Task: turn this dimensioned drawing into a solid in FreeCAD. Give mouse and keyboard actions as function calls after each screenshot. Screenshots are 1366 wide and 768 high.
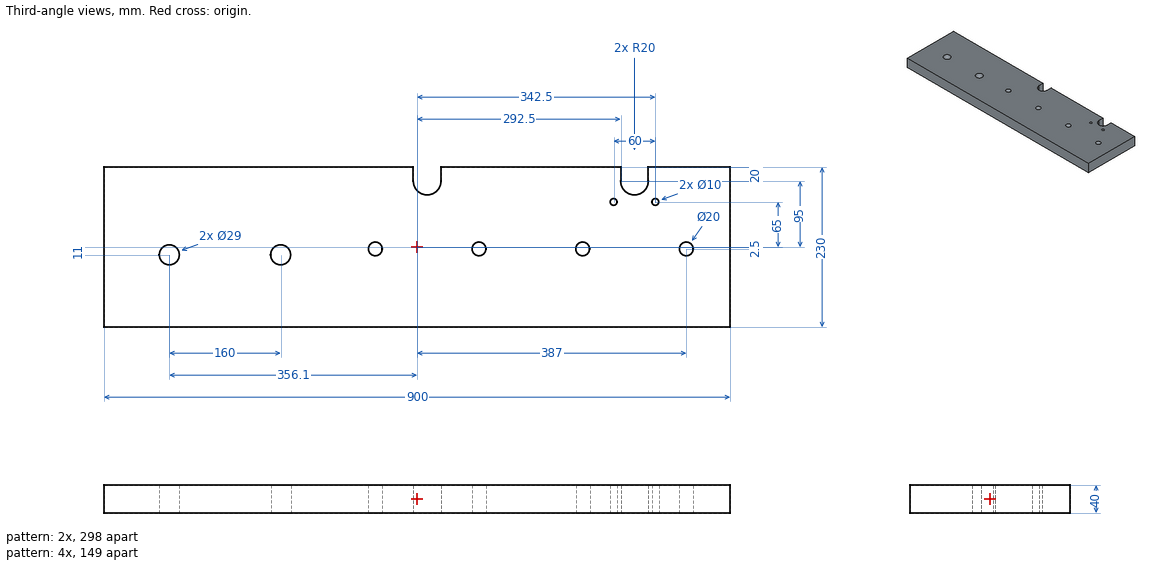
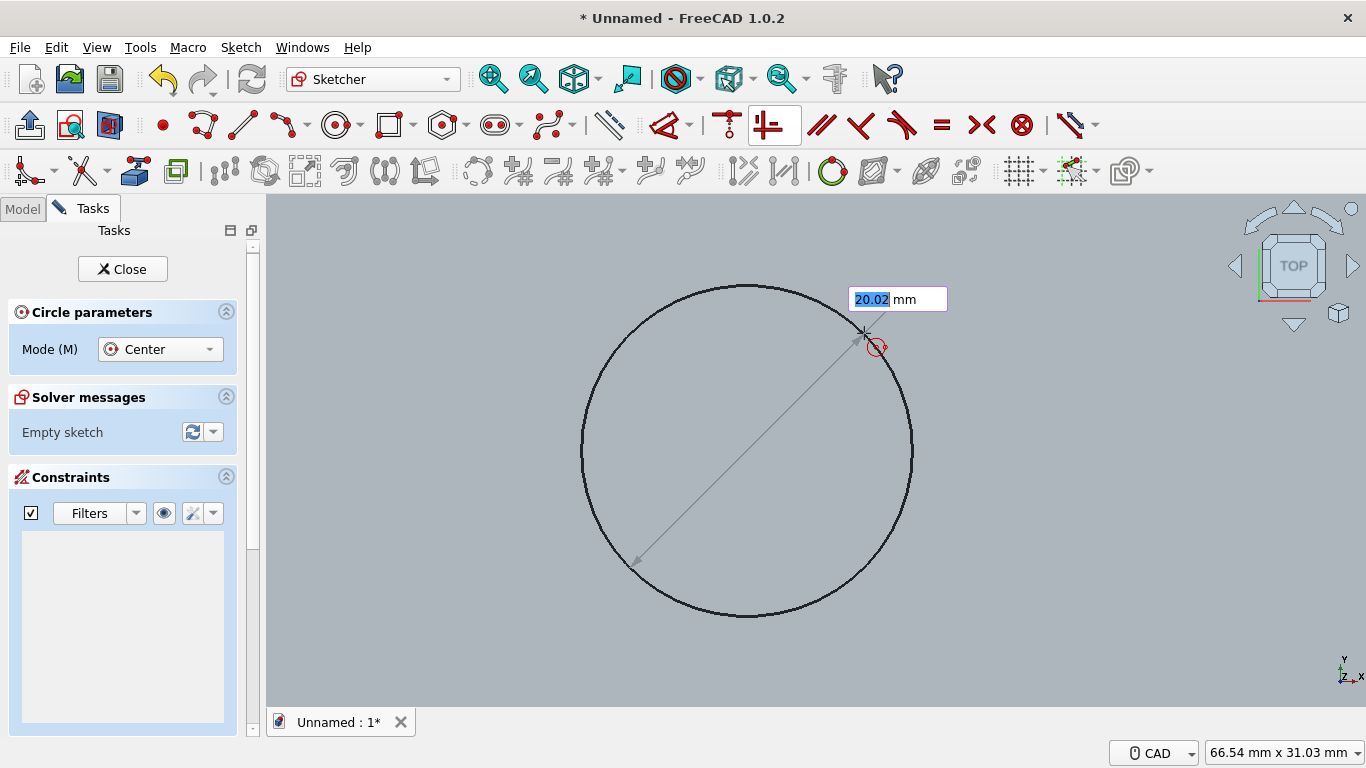
text(20)
key(Return)
key(Escape)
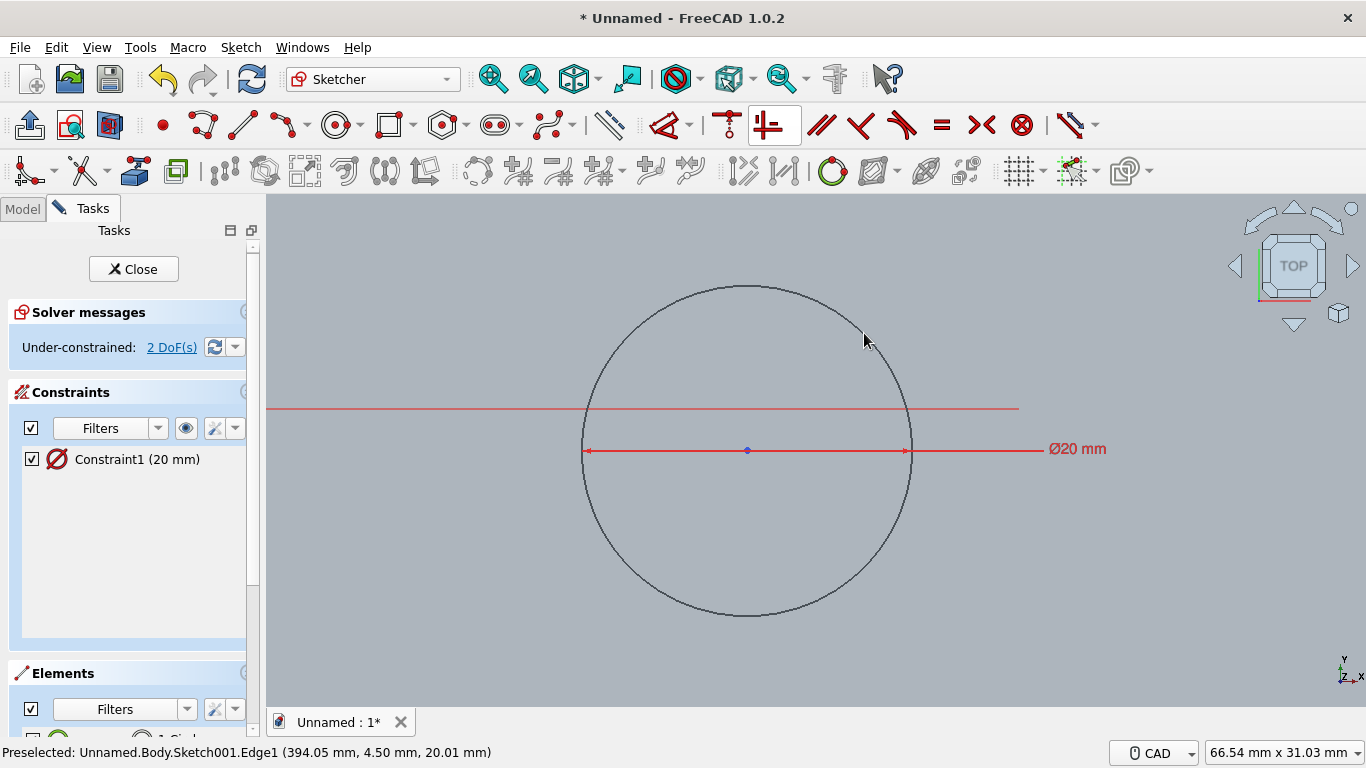
click(747, 451)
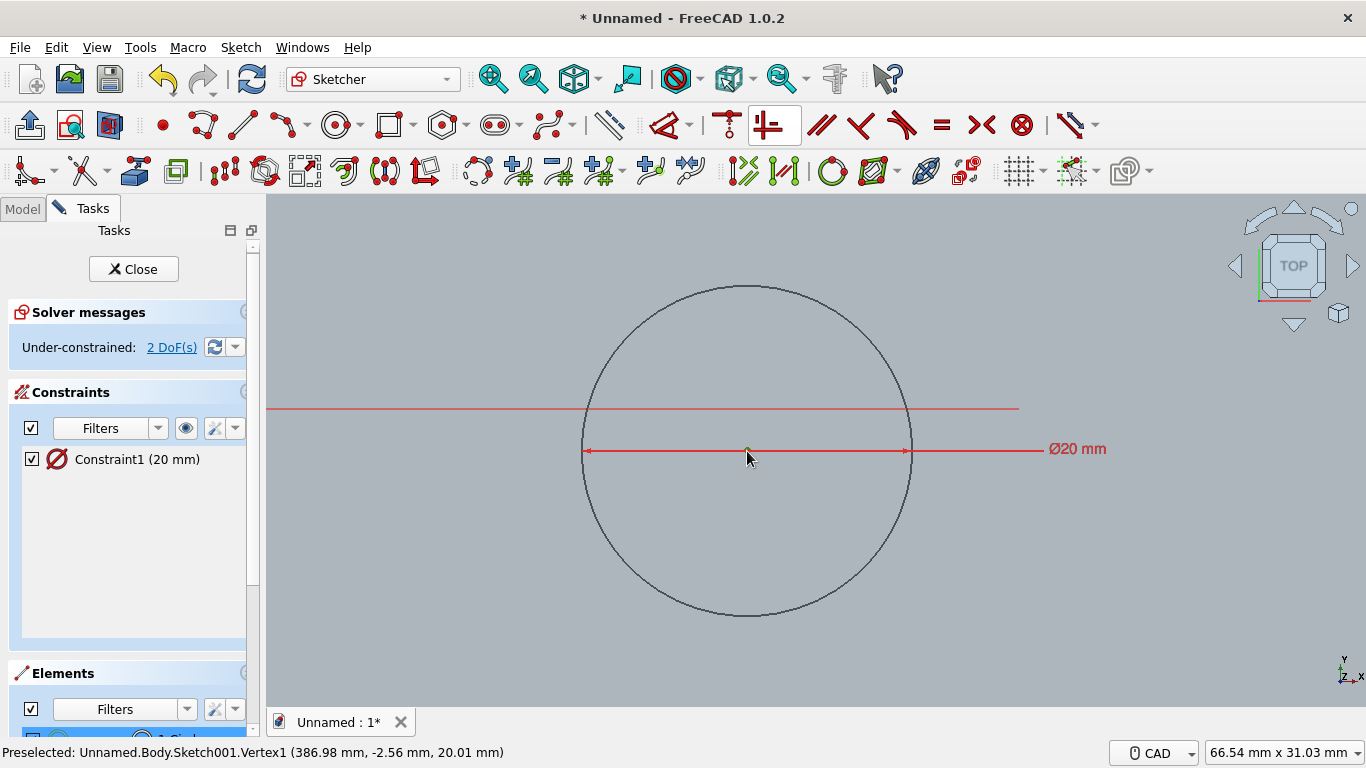
click(692, 126)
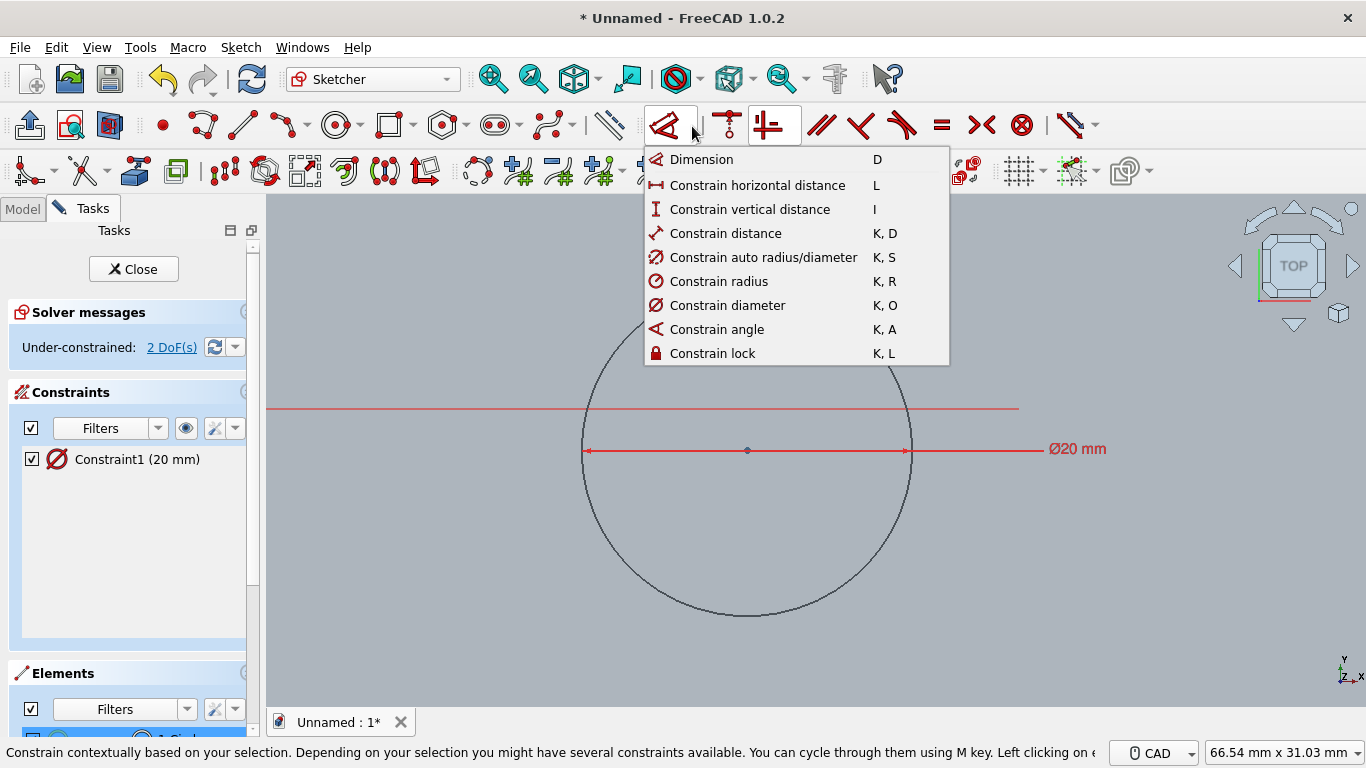
click(797, 185)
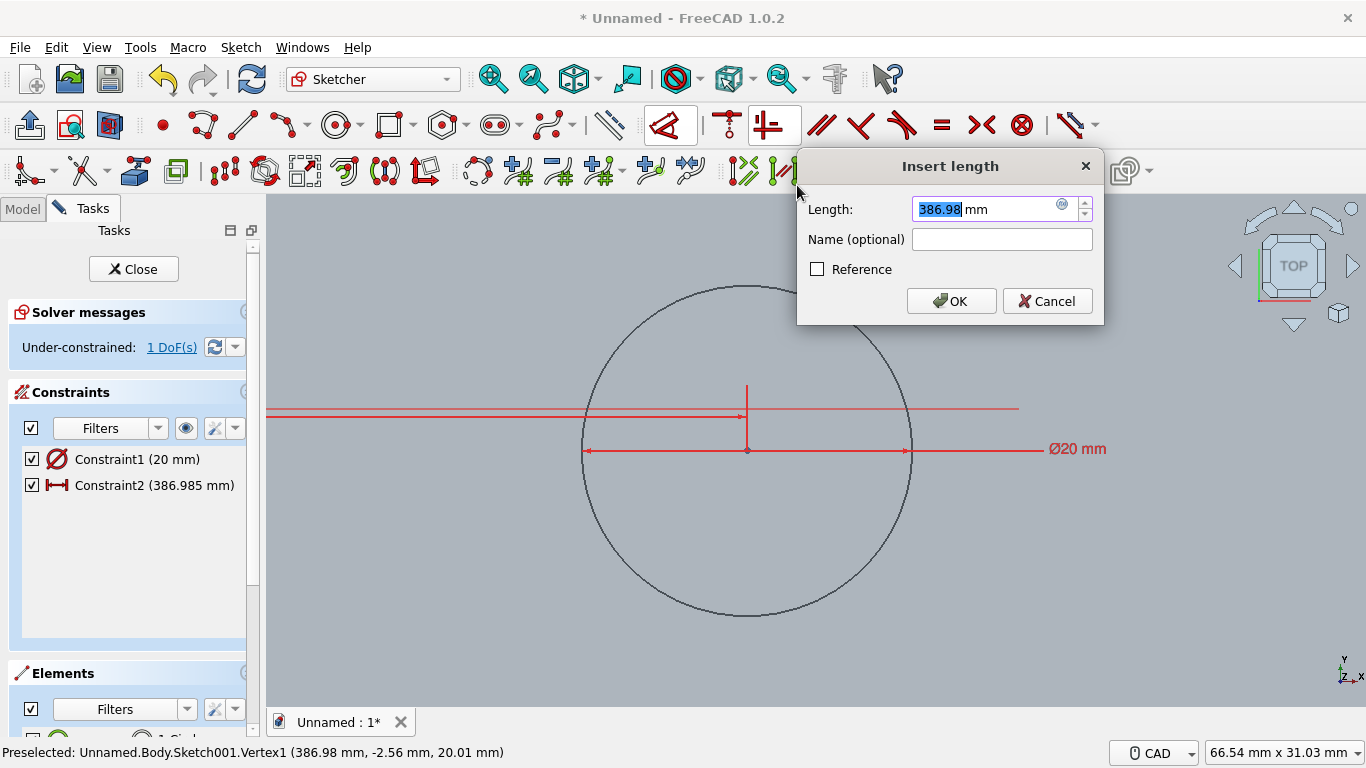
text(387)
key(Return)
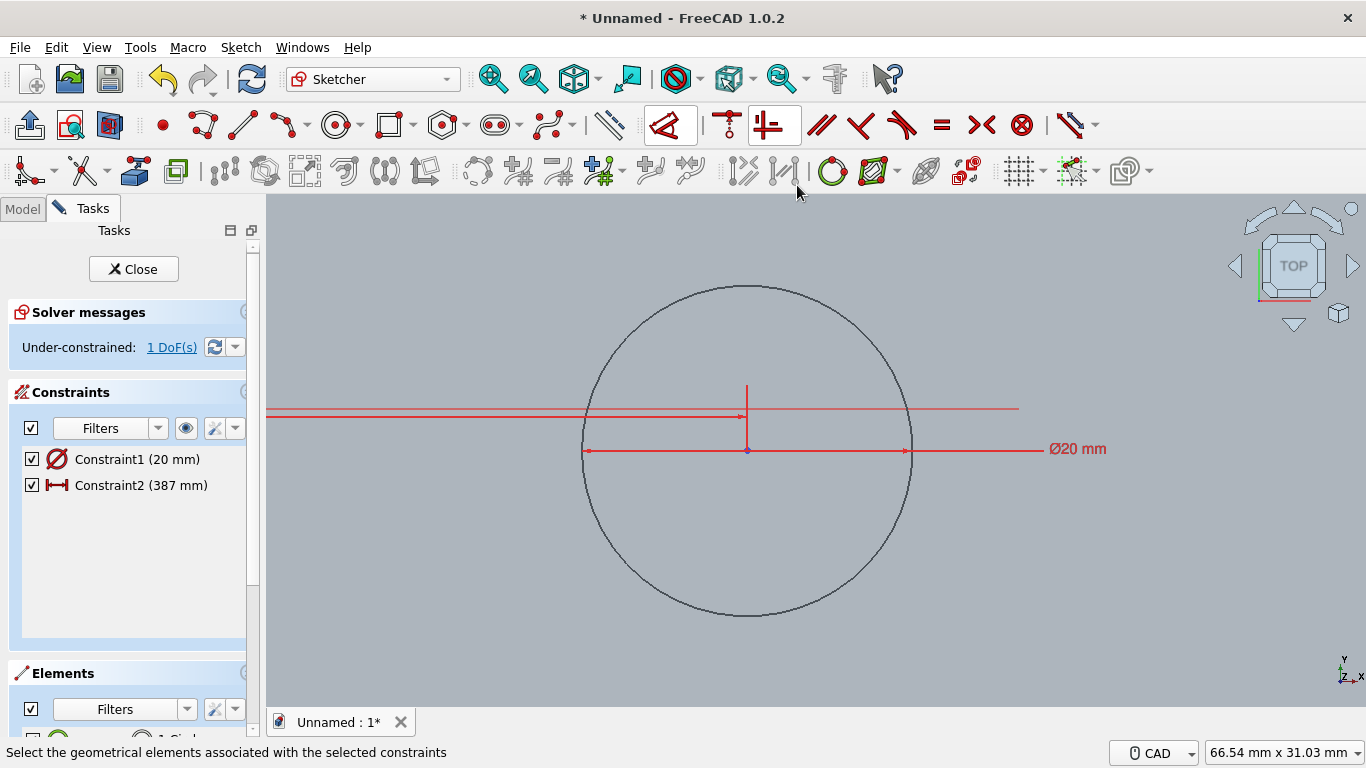
click(747, 451)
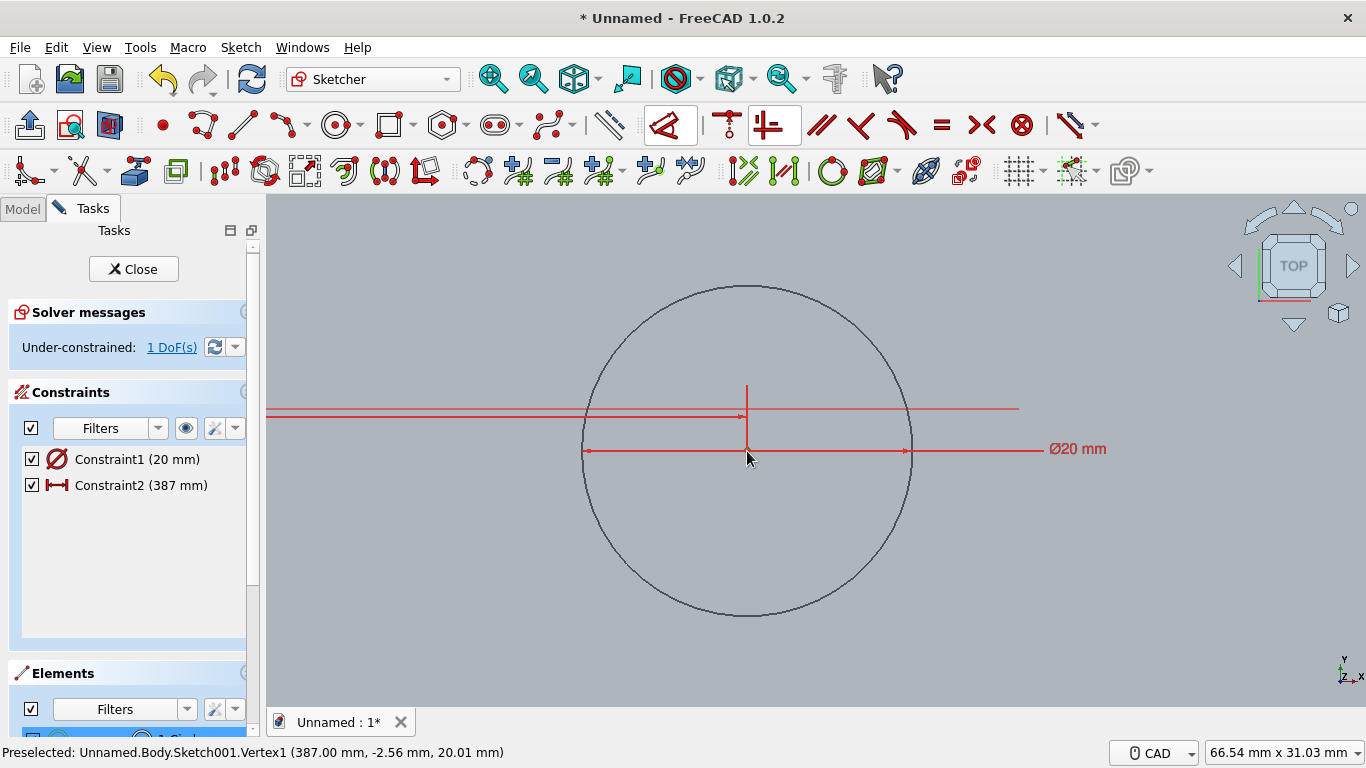
key(i)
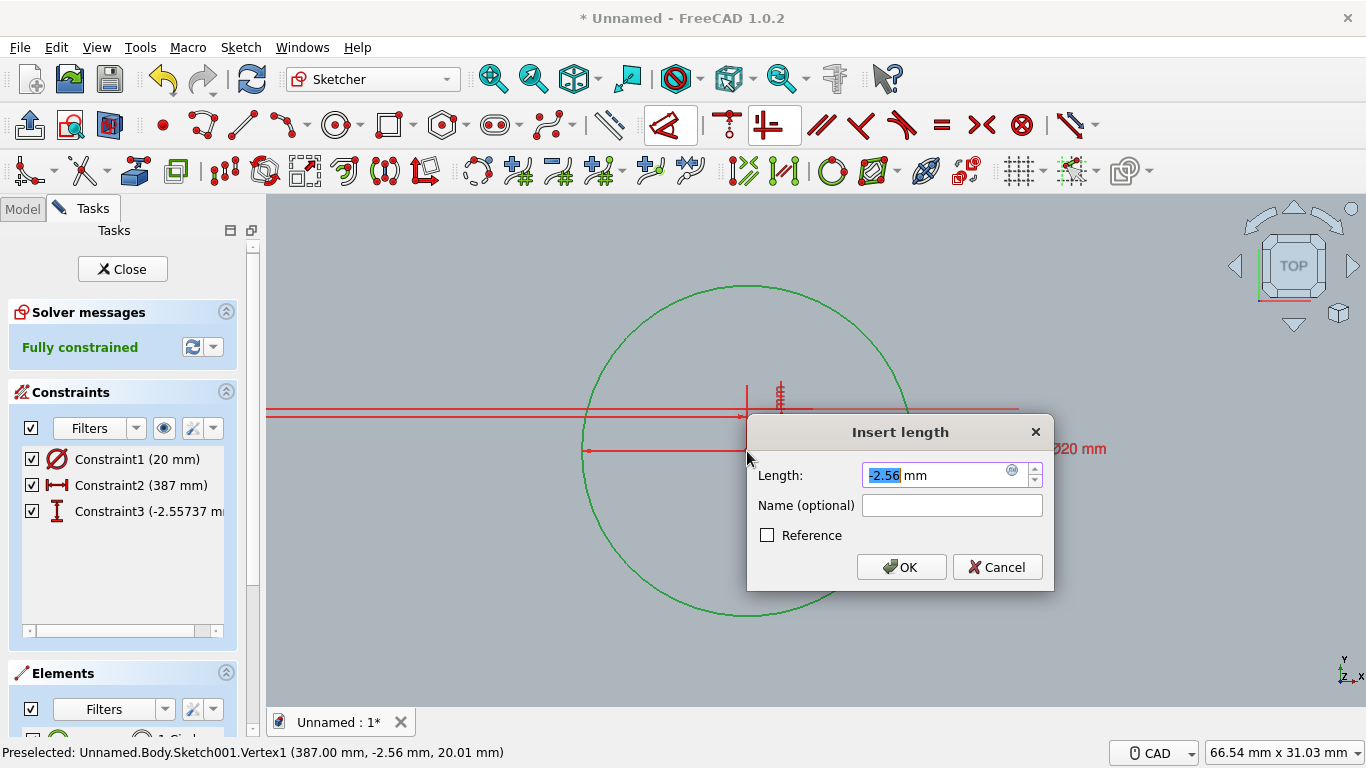
text(-2.5)
key(Return)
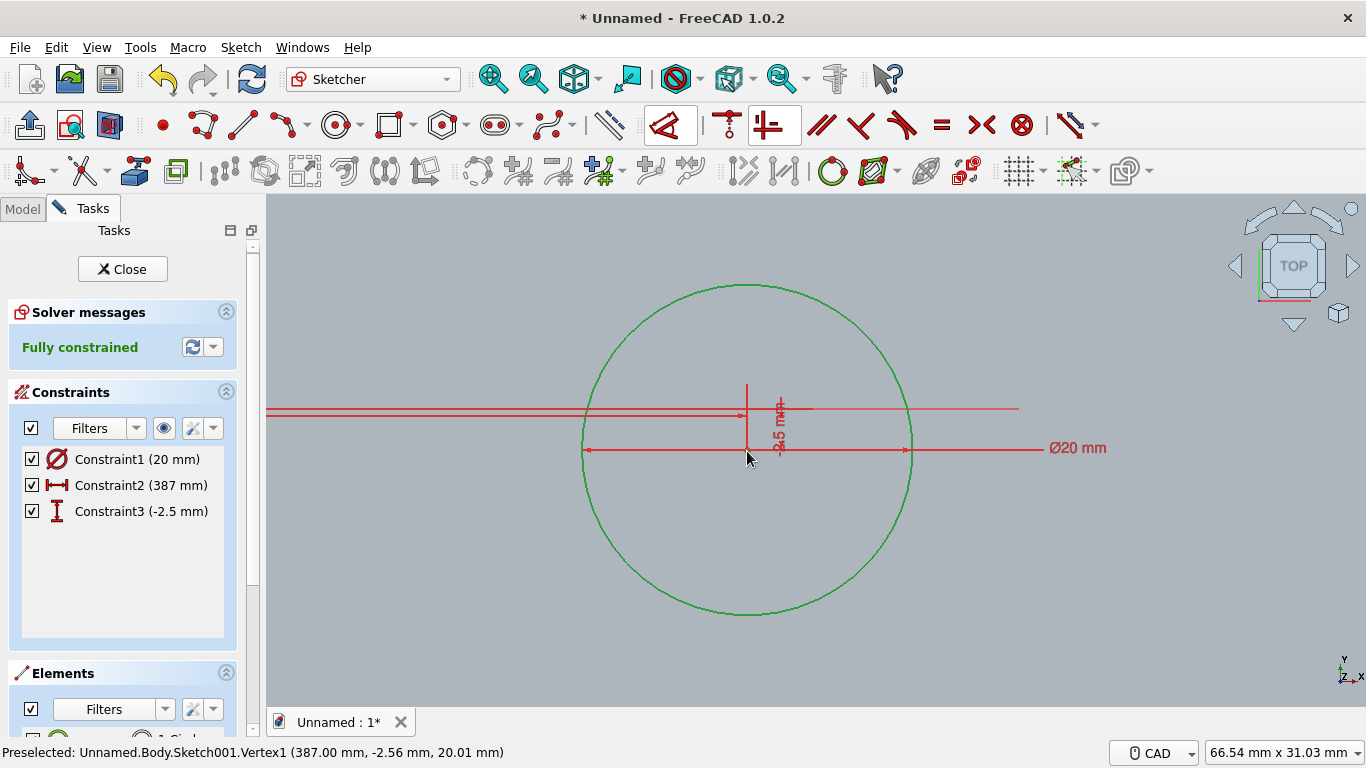
click(123, 269)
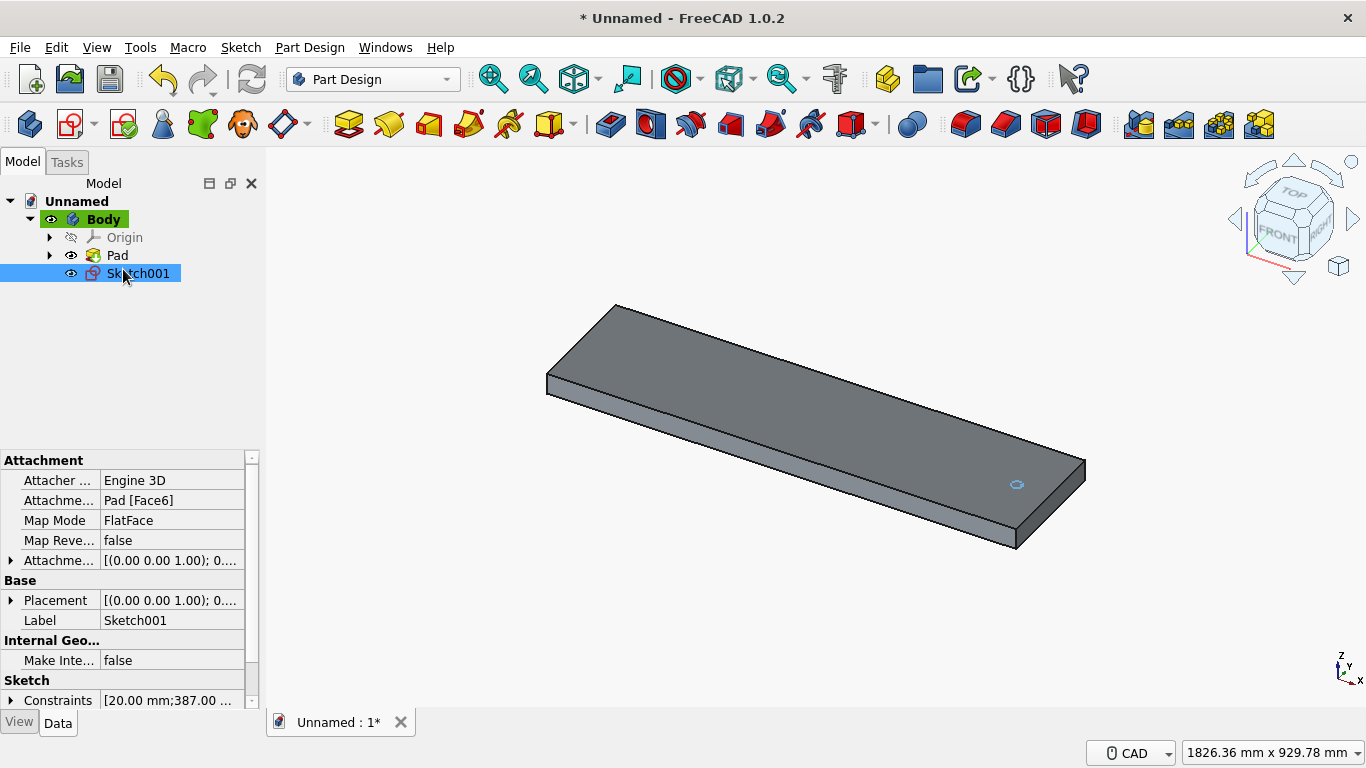
click(612, 124)